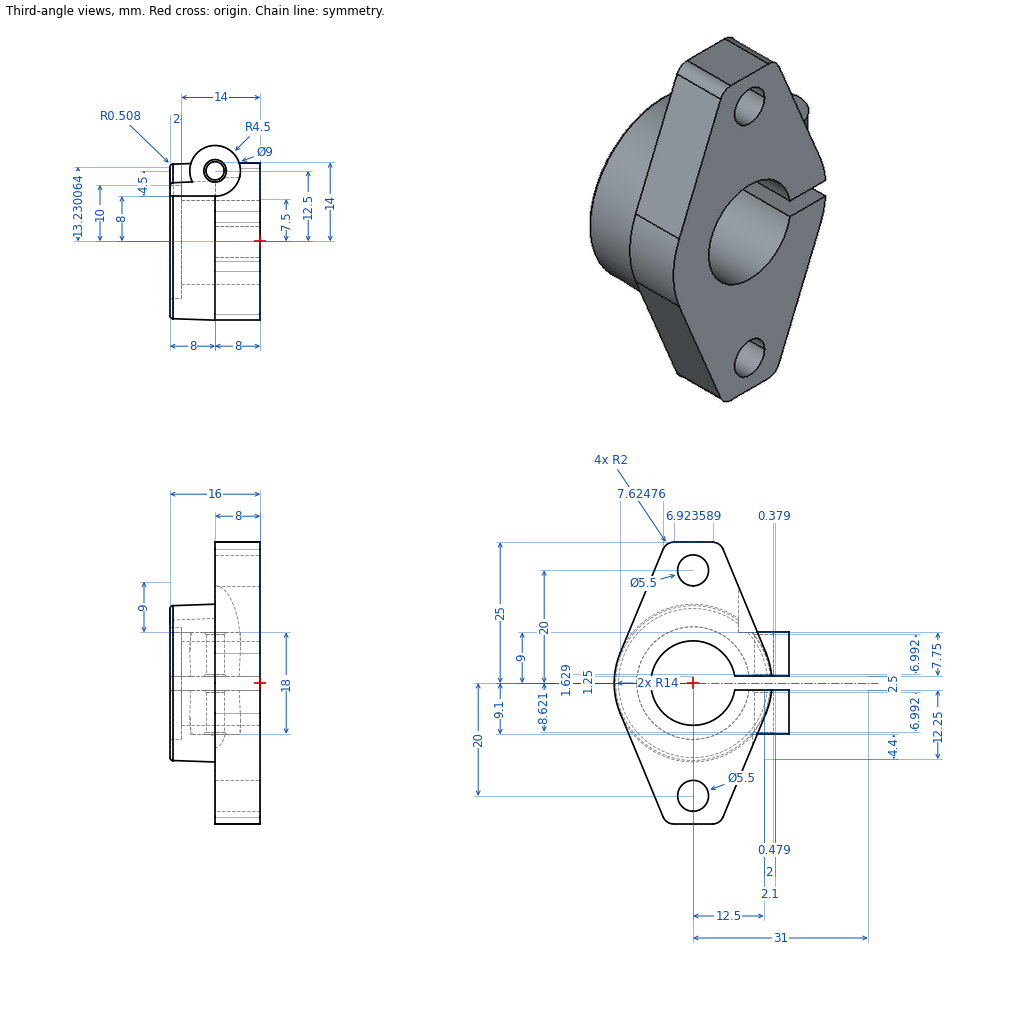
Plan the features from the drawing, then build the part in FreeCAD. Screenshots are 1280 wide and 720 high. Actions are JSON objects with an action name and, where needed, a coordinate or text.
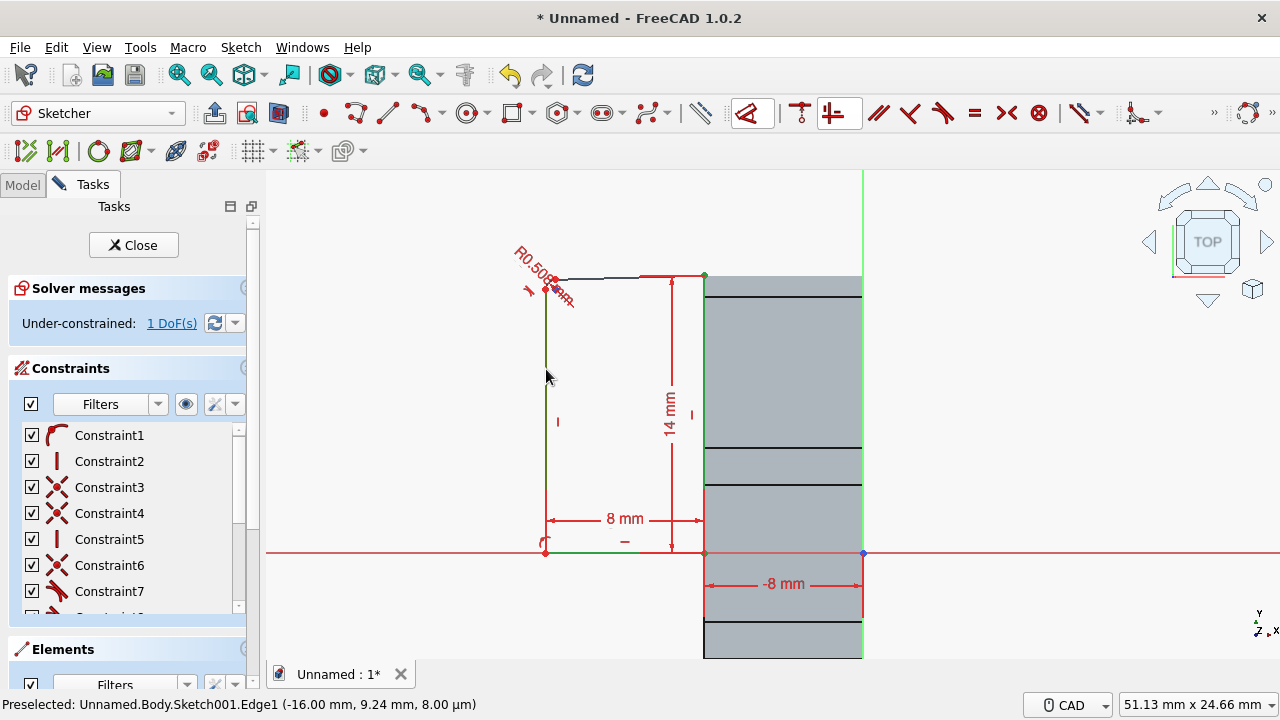
{"action": "left_click", "coordinate": [768, 114]}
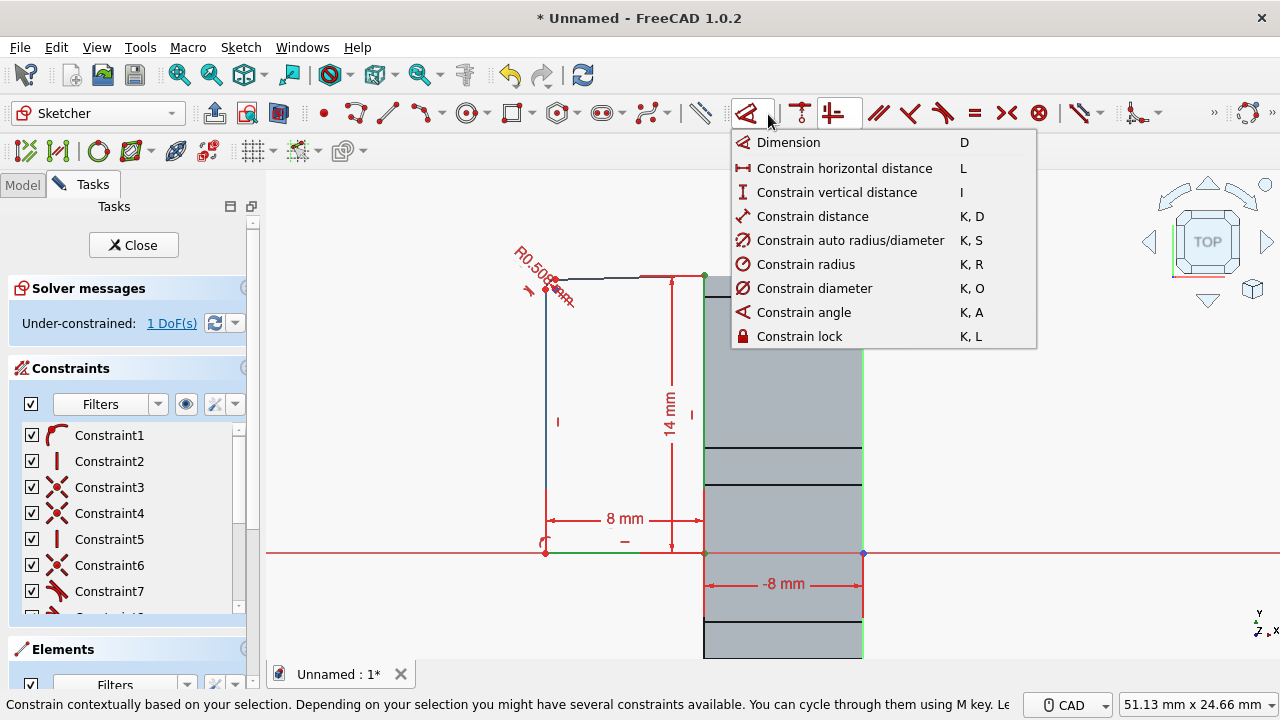
{"action": "left_click", "coordinate": [884, 192]}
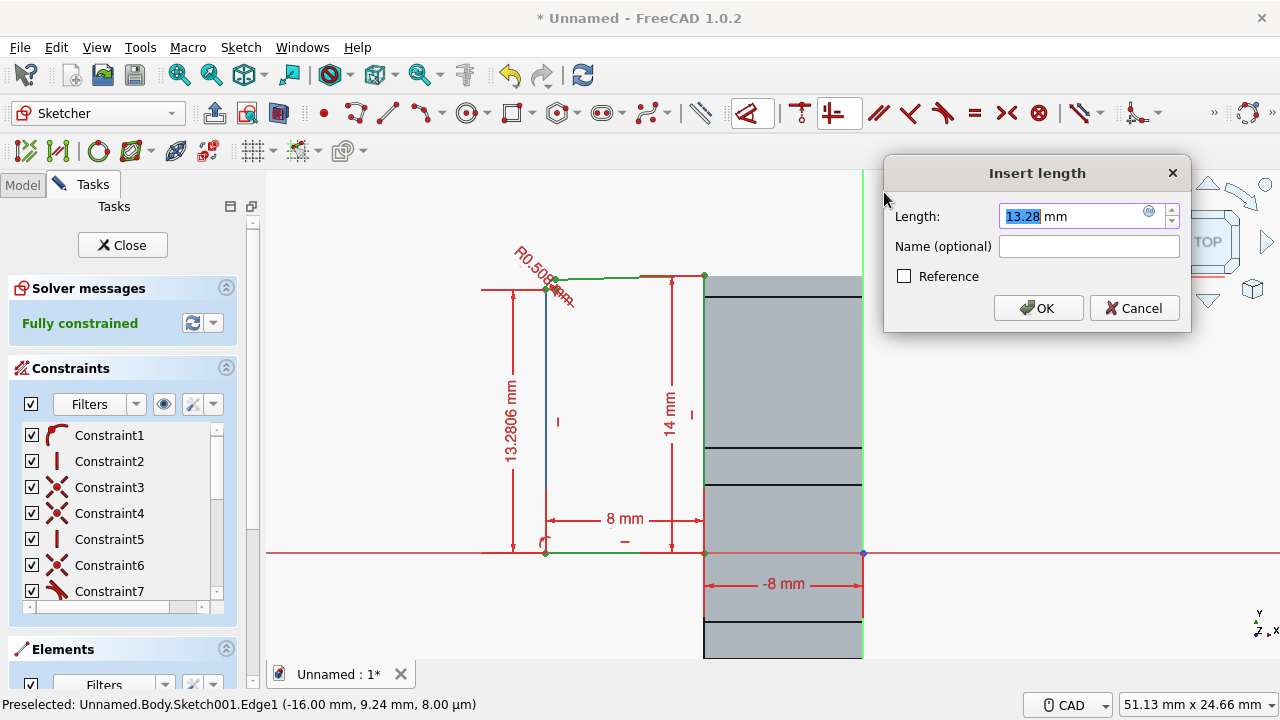
{"action": "type", "text": "13.230064"}
{"action": "key", "text": "Return"}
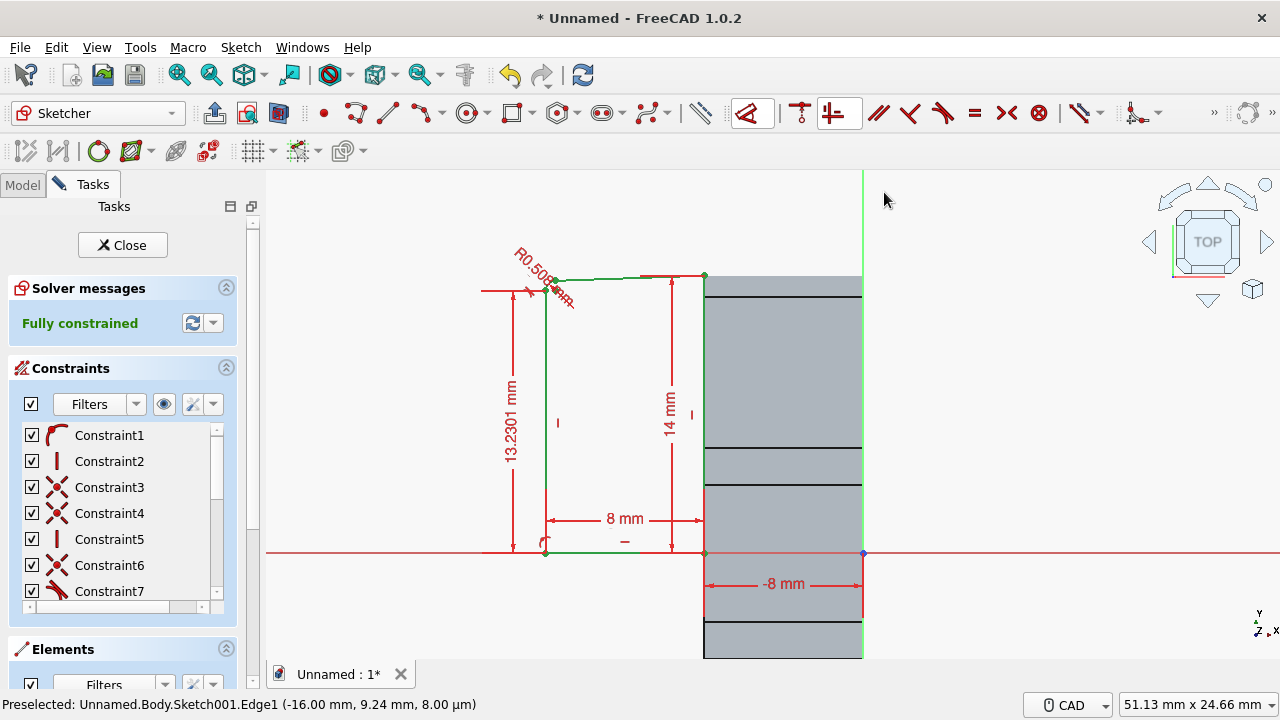
{"action": "left_click", "coordinate": [123, 245]}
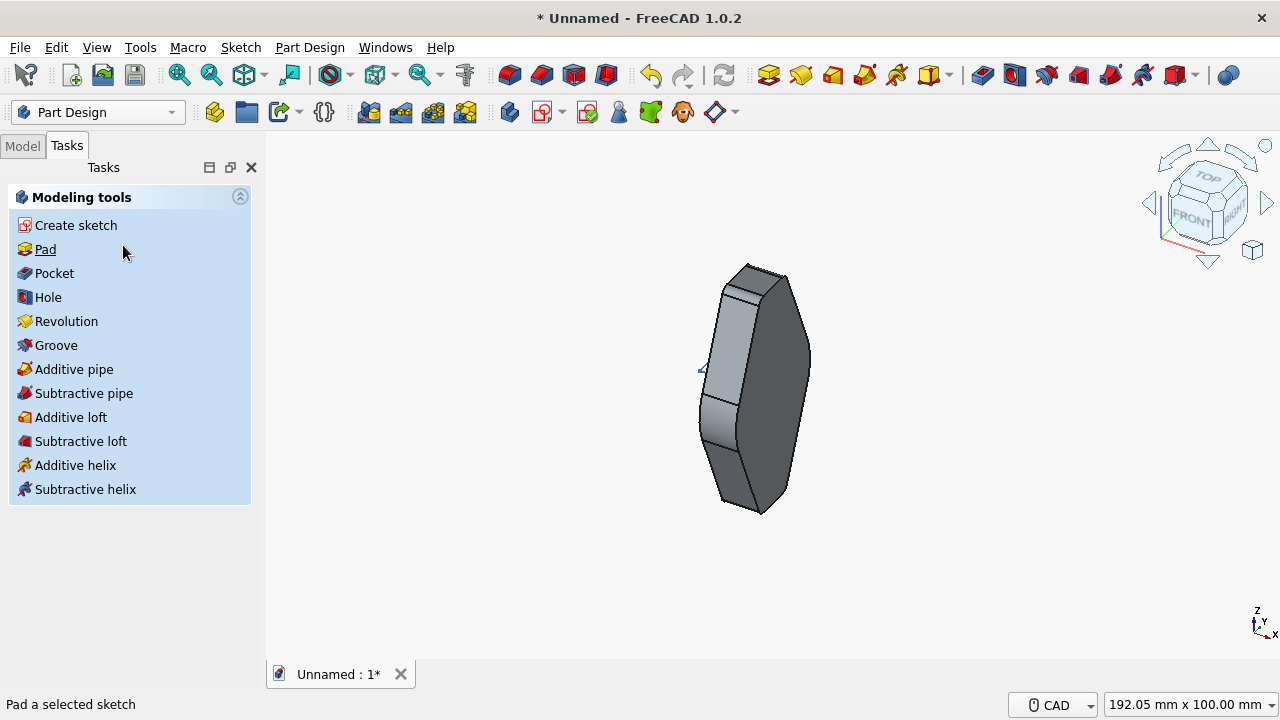
{"action": "left_click", "coordinate": [802, 76]}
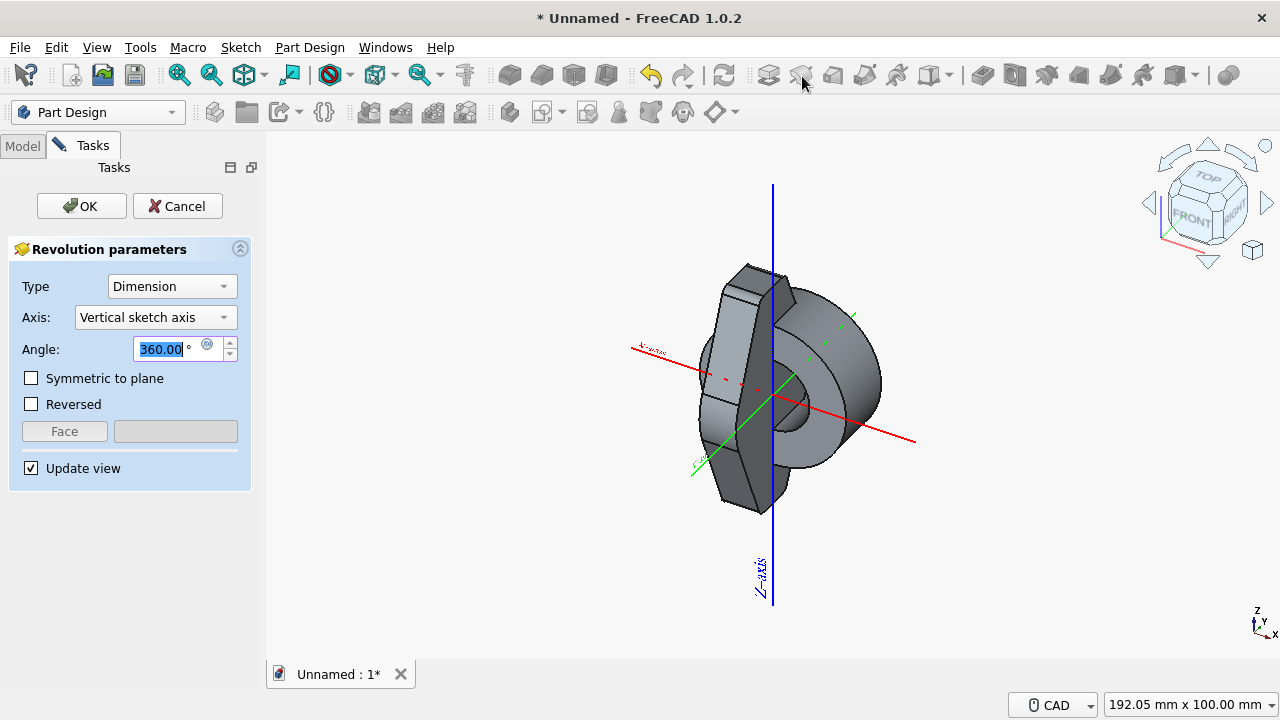
{"action": "left_click", "coordinate": [156, 318]}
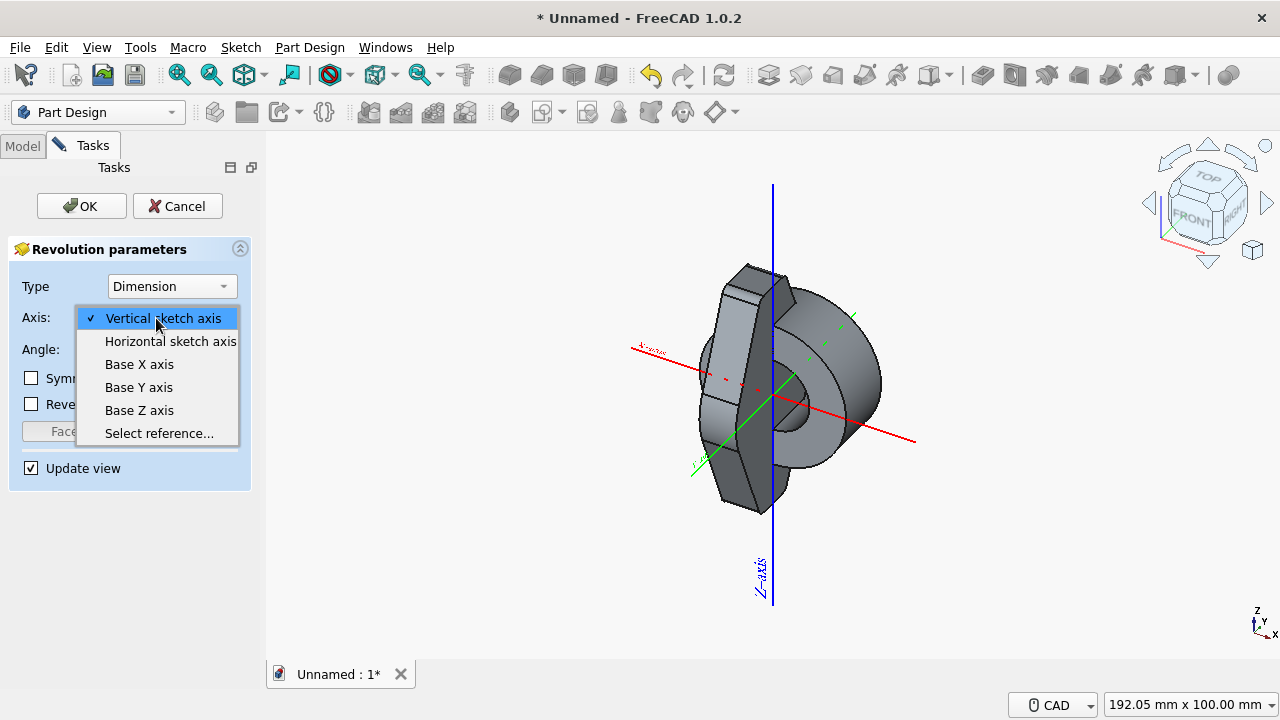
{"action": "left_click", "coordinate": [156, 342]}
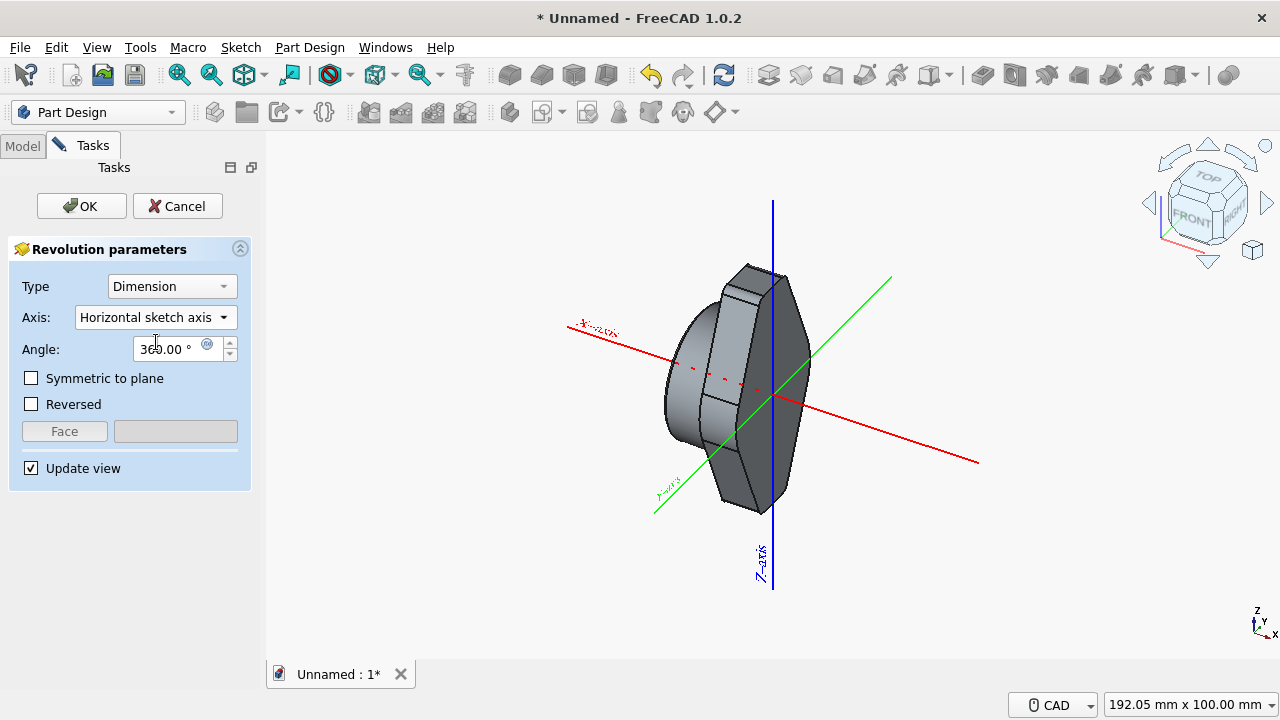
{"action": "left_click", "coordinate": [82, 206]}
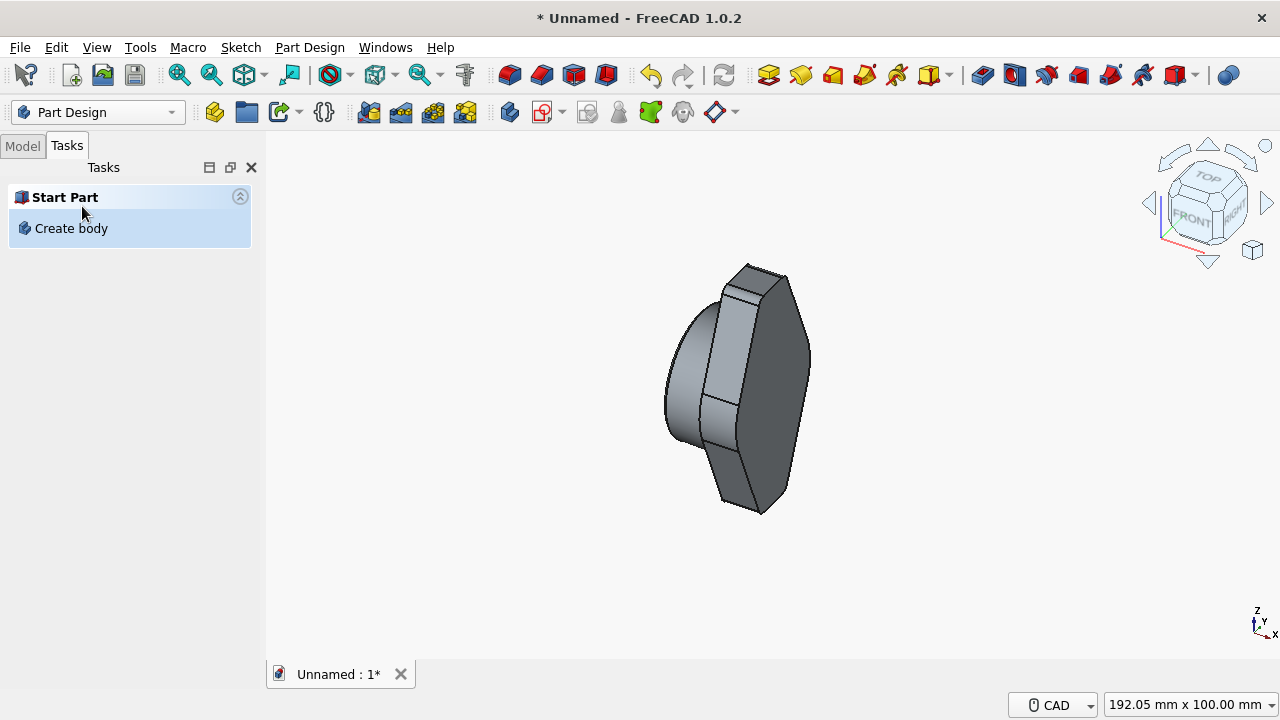
{"action": "left_click", "coordinate": [542, 112]}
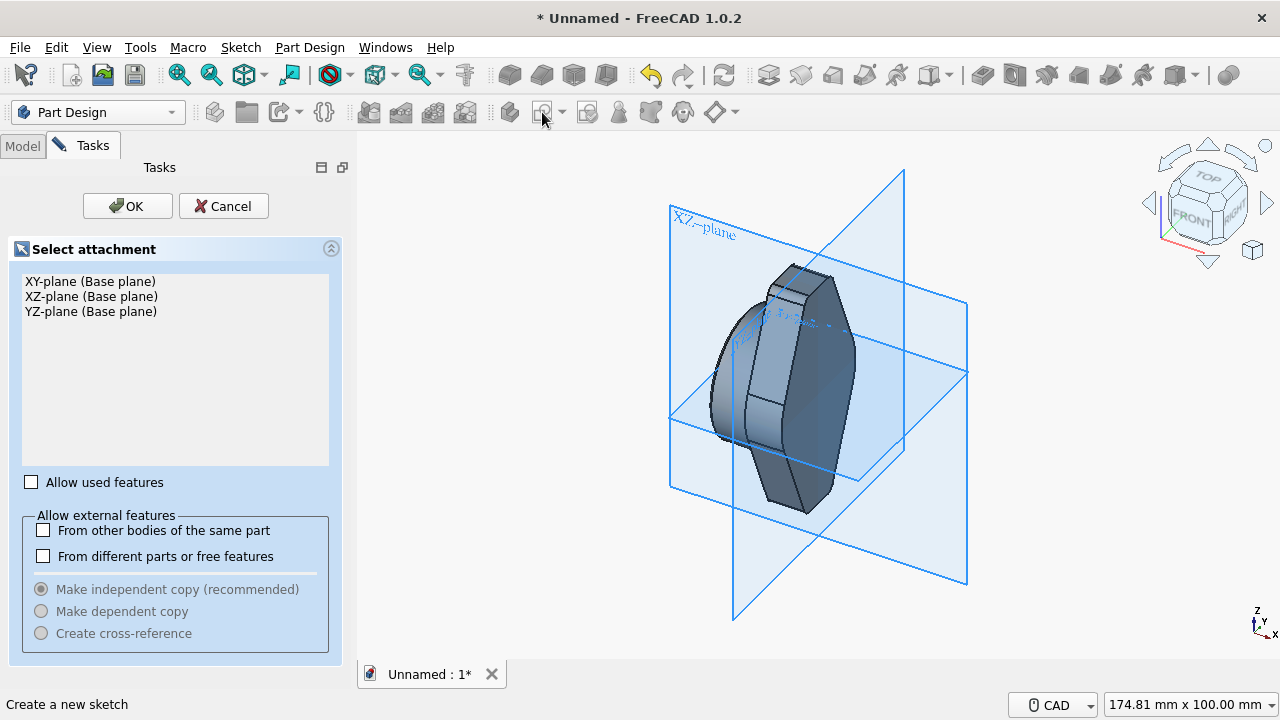
{"action": "left_click", "coordinate": [82, 282]}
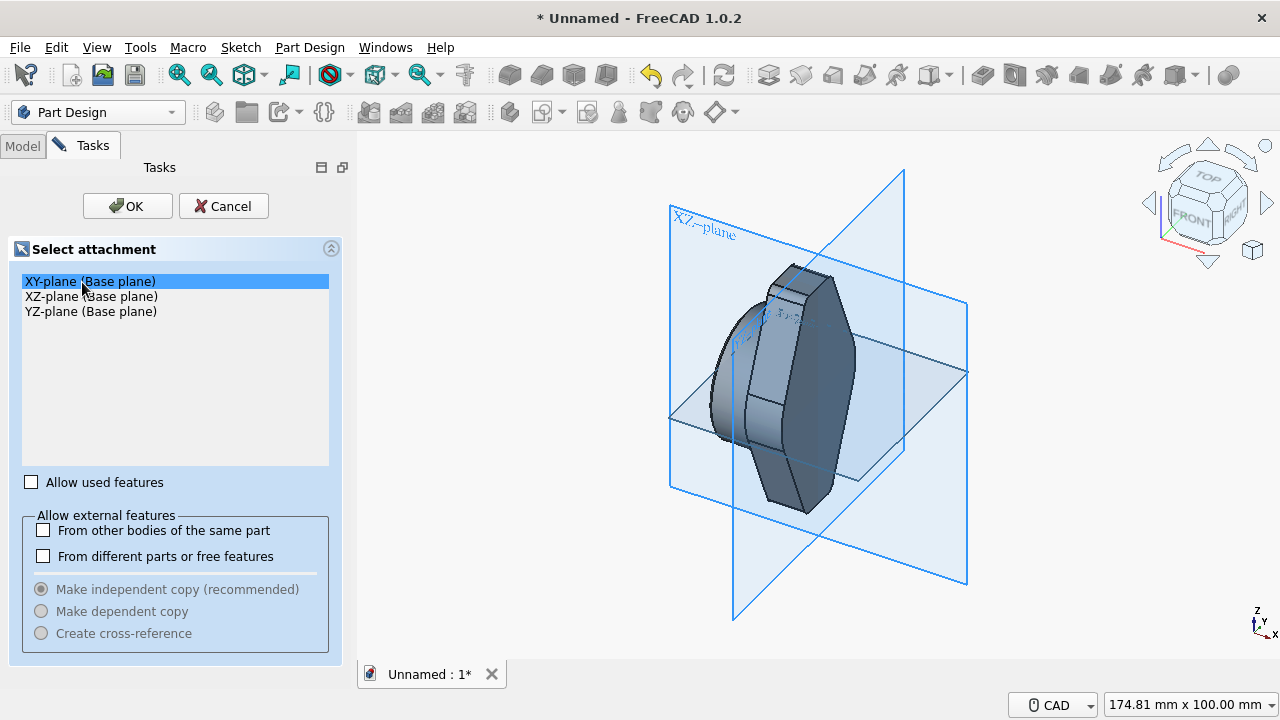
{"action": "left_click", "coordinate": [128, 206]}